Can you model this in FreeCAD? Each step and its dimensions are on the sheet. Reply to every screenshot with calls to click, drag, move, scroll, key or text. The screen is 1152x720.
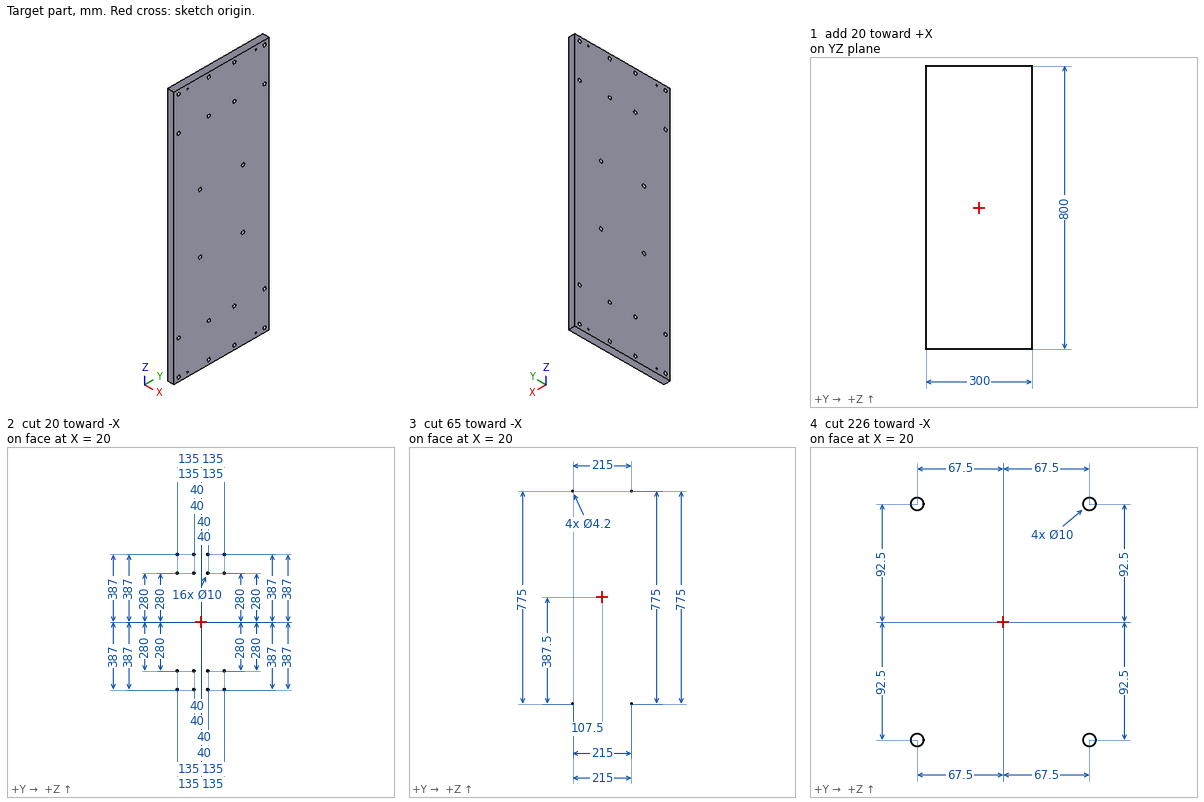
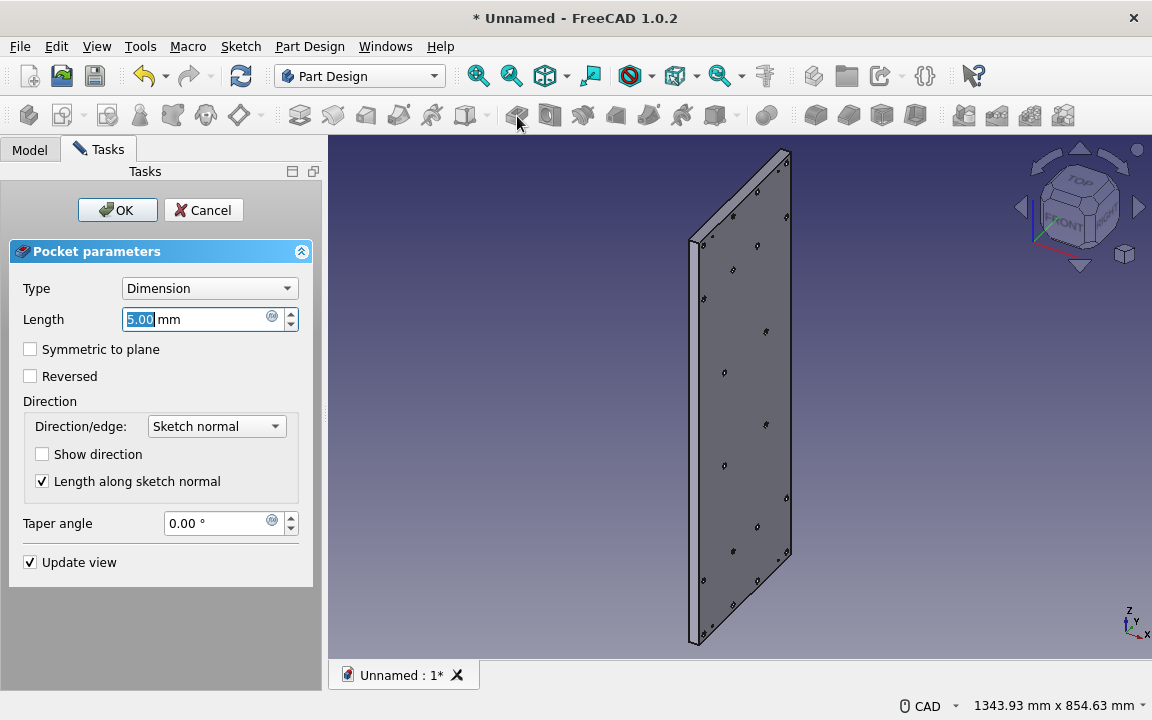
text(226)
key(Tab)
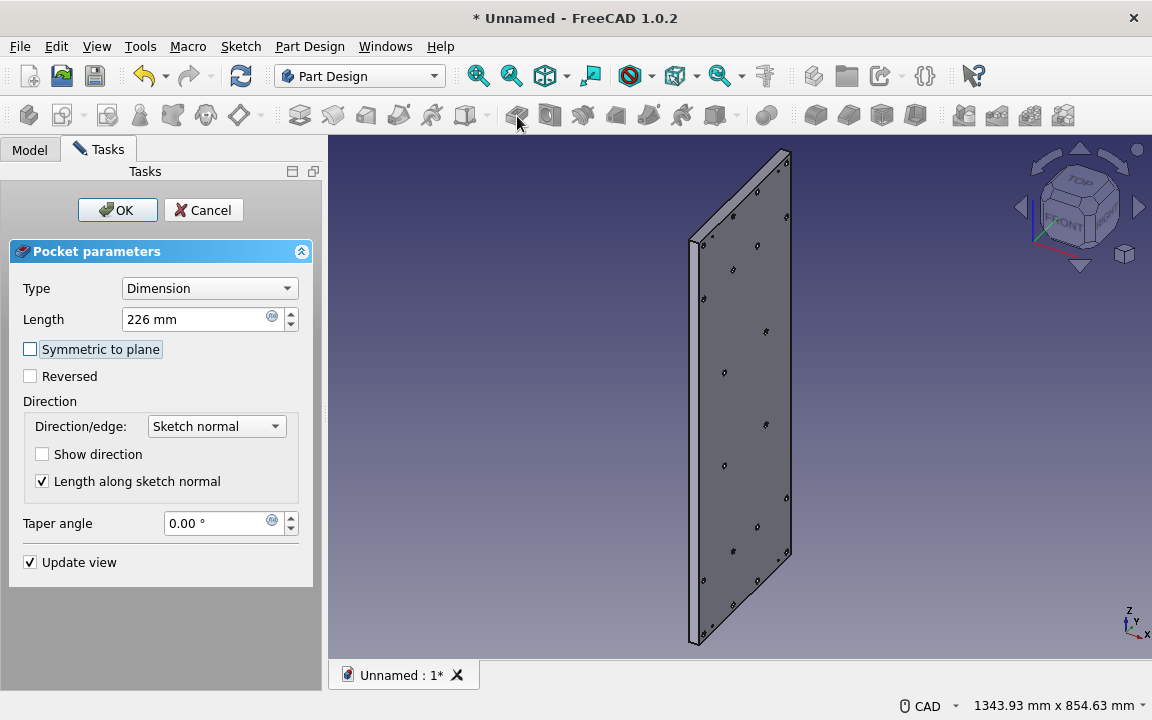
click(118, 210)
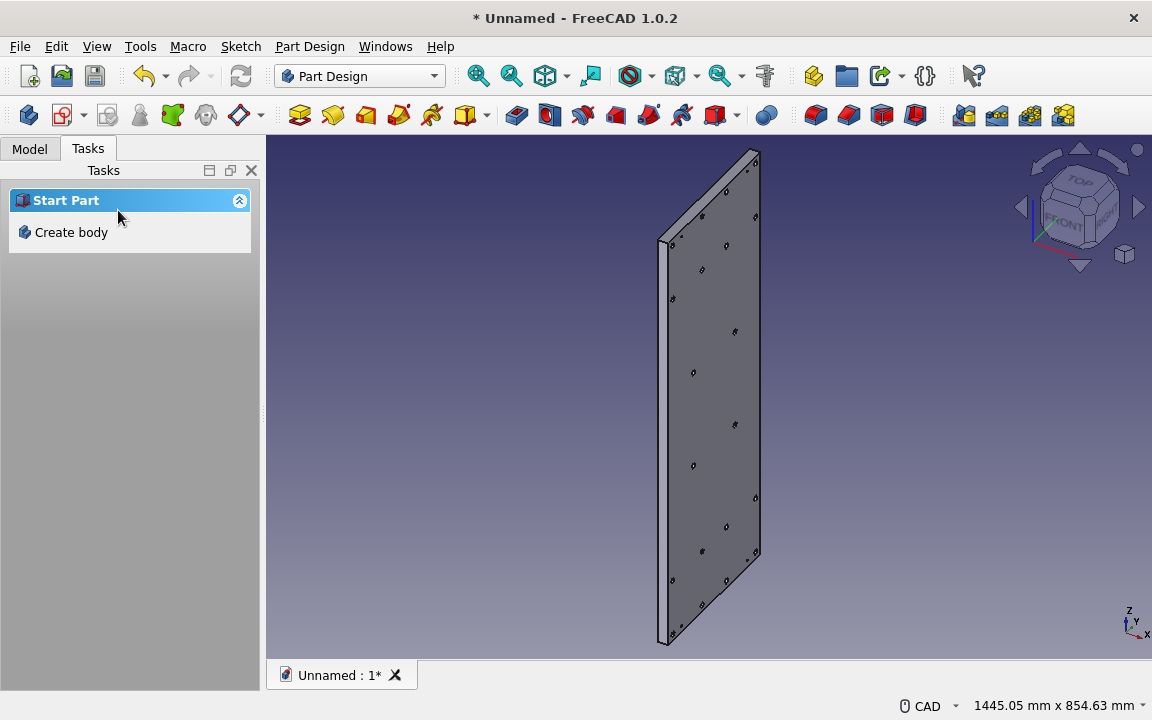
key(0)